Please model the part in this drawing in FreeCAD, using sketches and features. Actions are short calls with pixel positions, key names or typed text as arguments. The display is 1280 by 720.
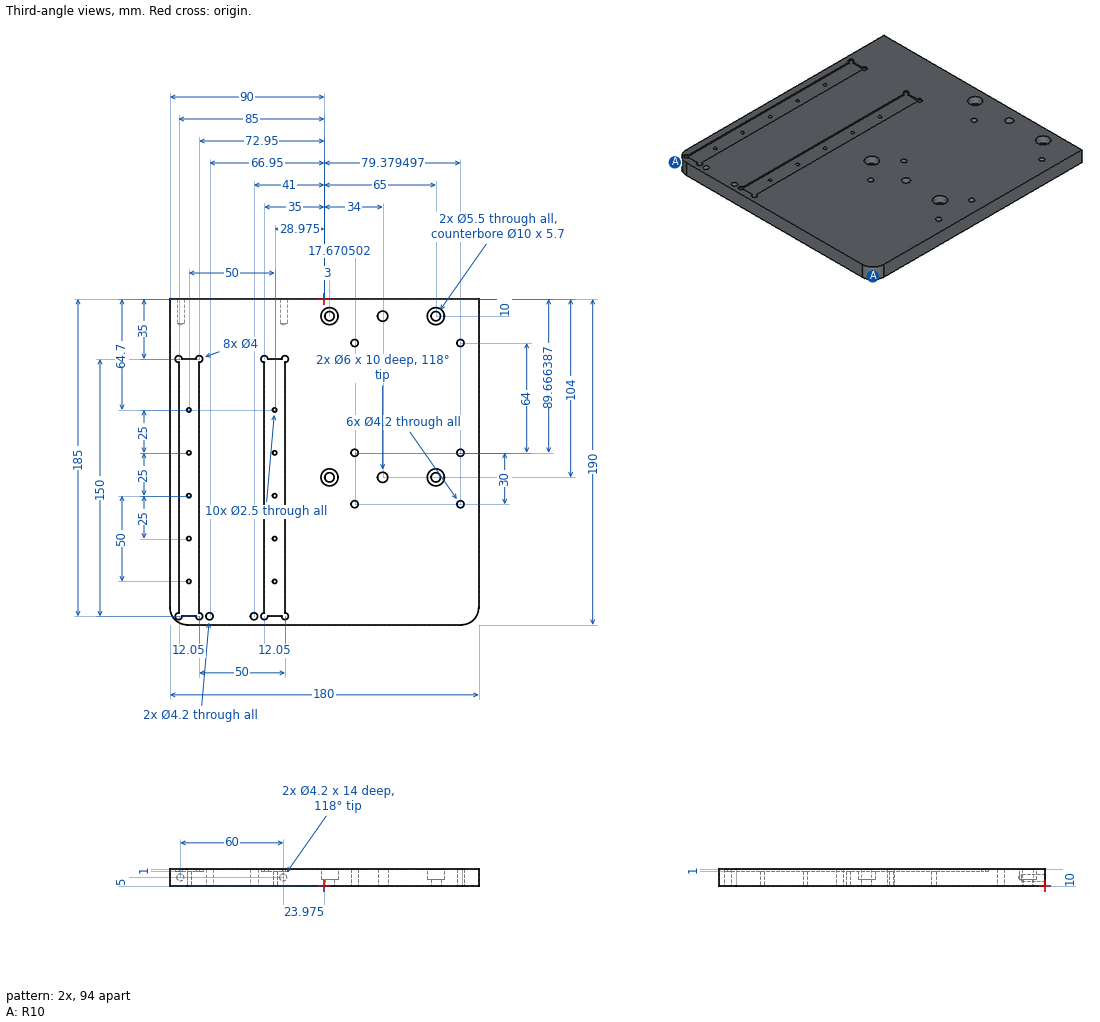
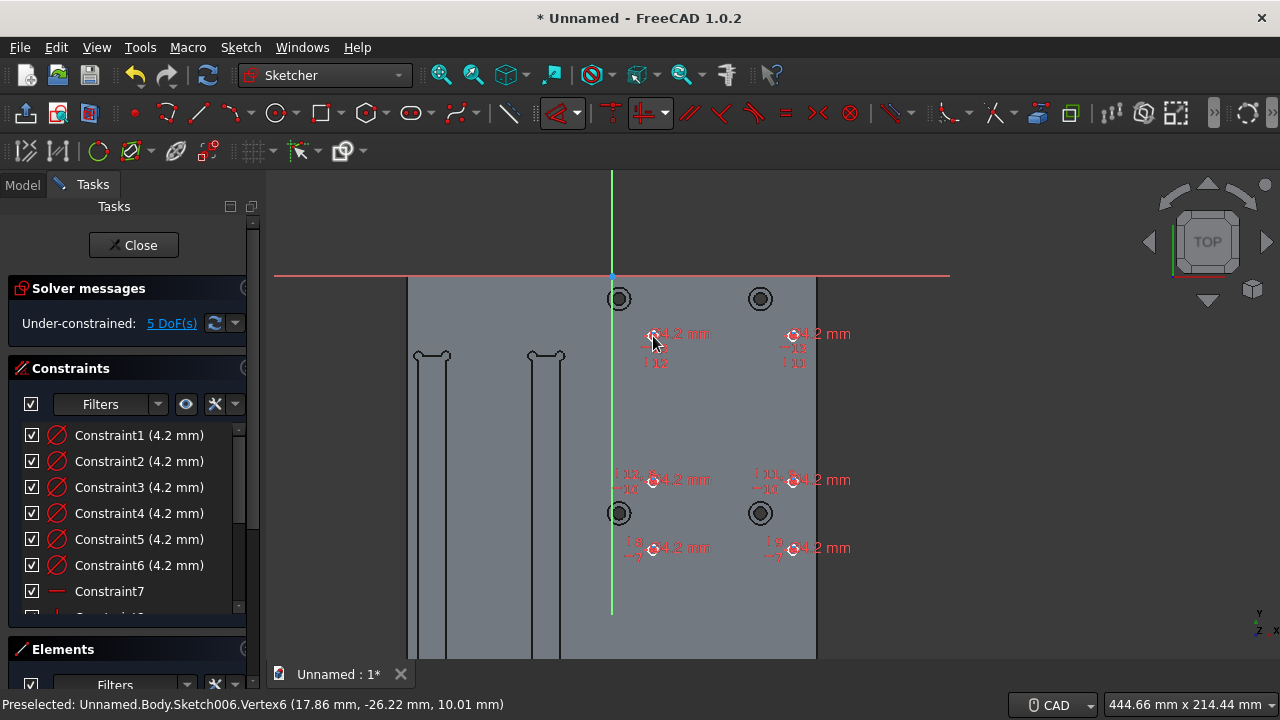
click(653, 550)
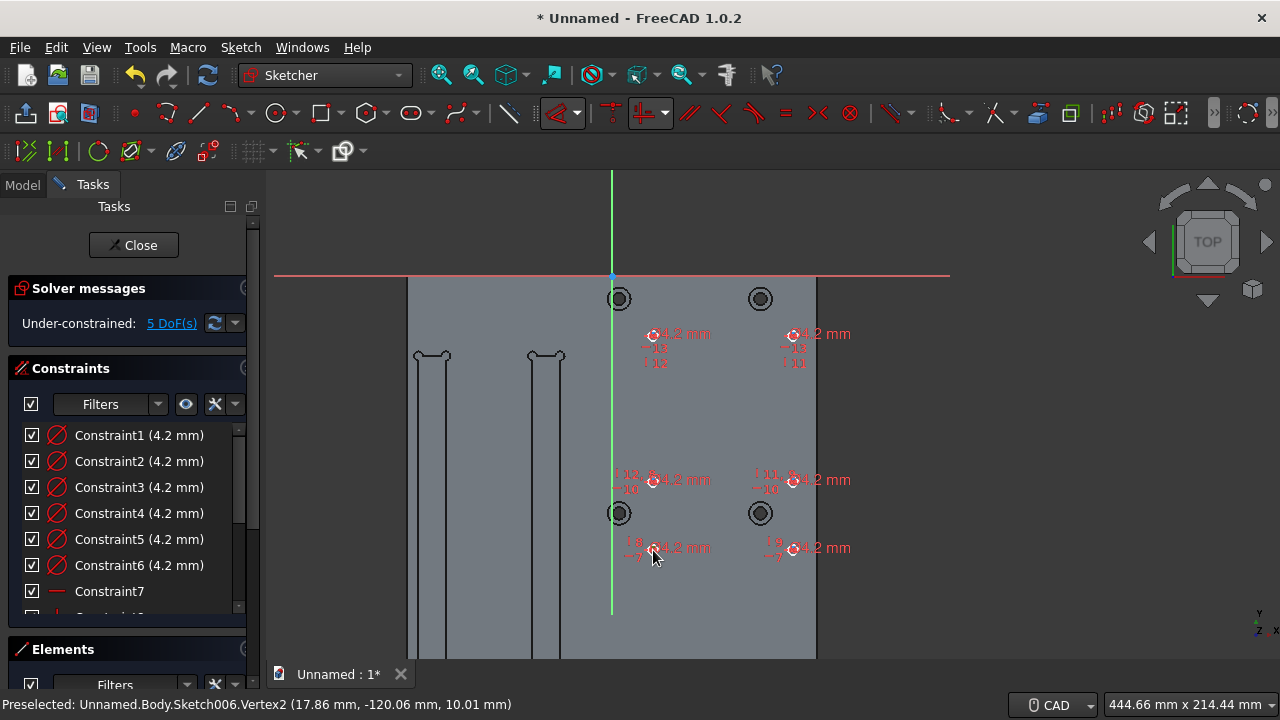
click(653, 482)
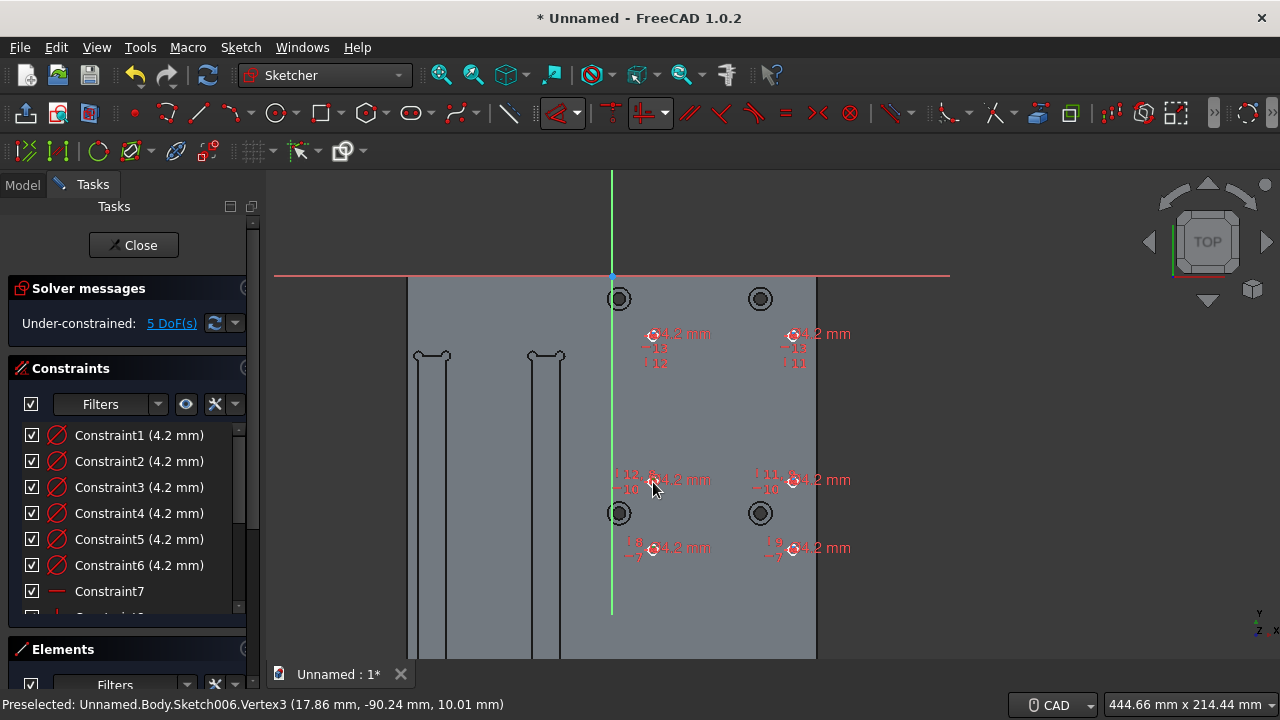
key(i)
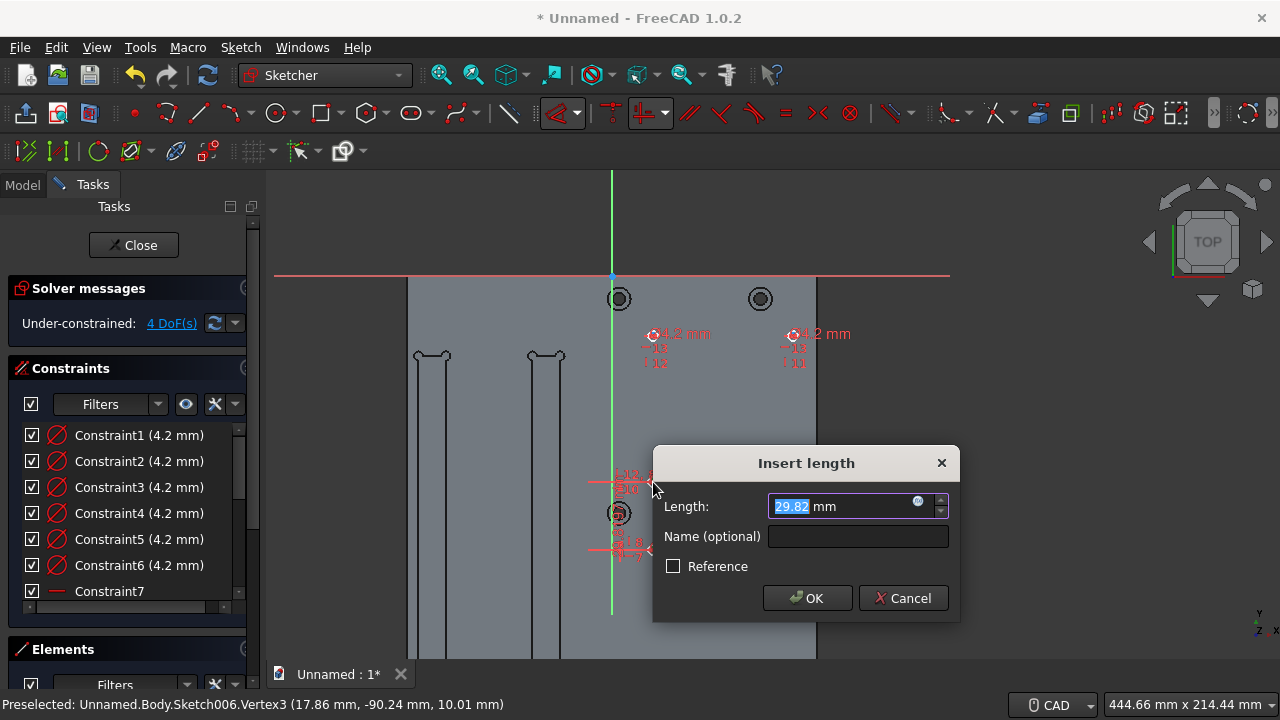
text(30)
key(Return)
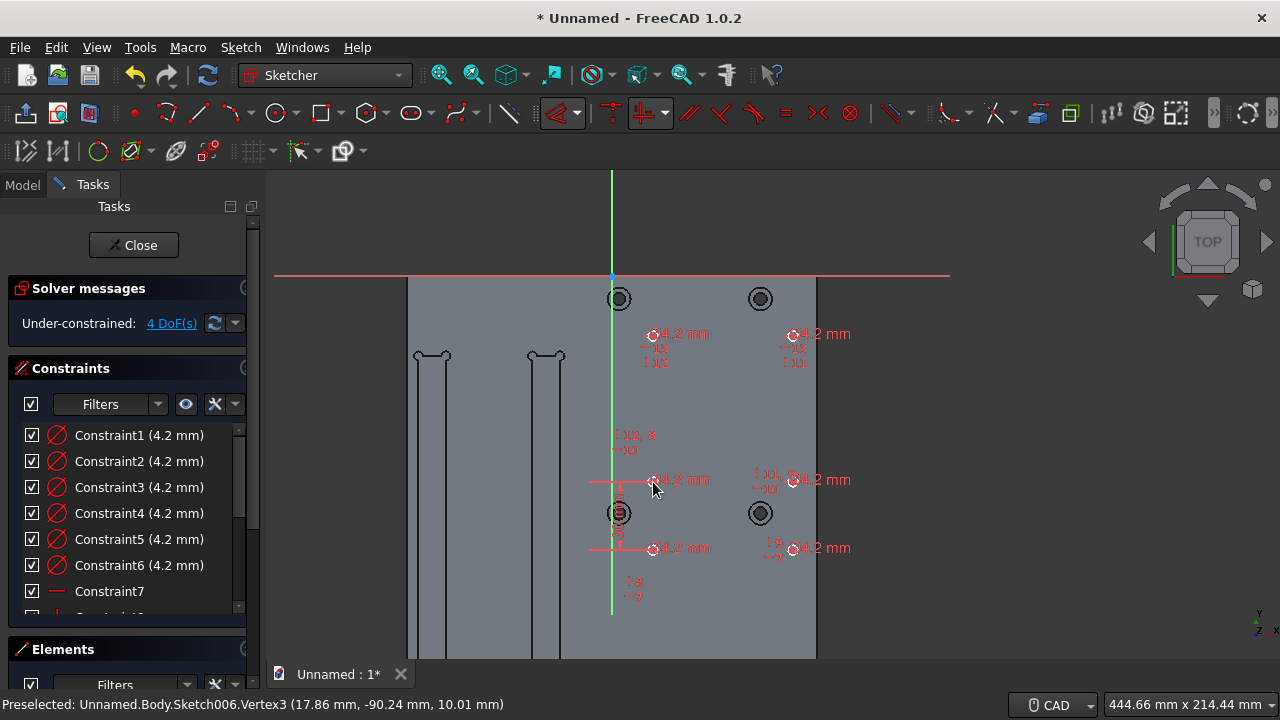
click(793, 482)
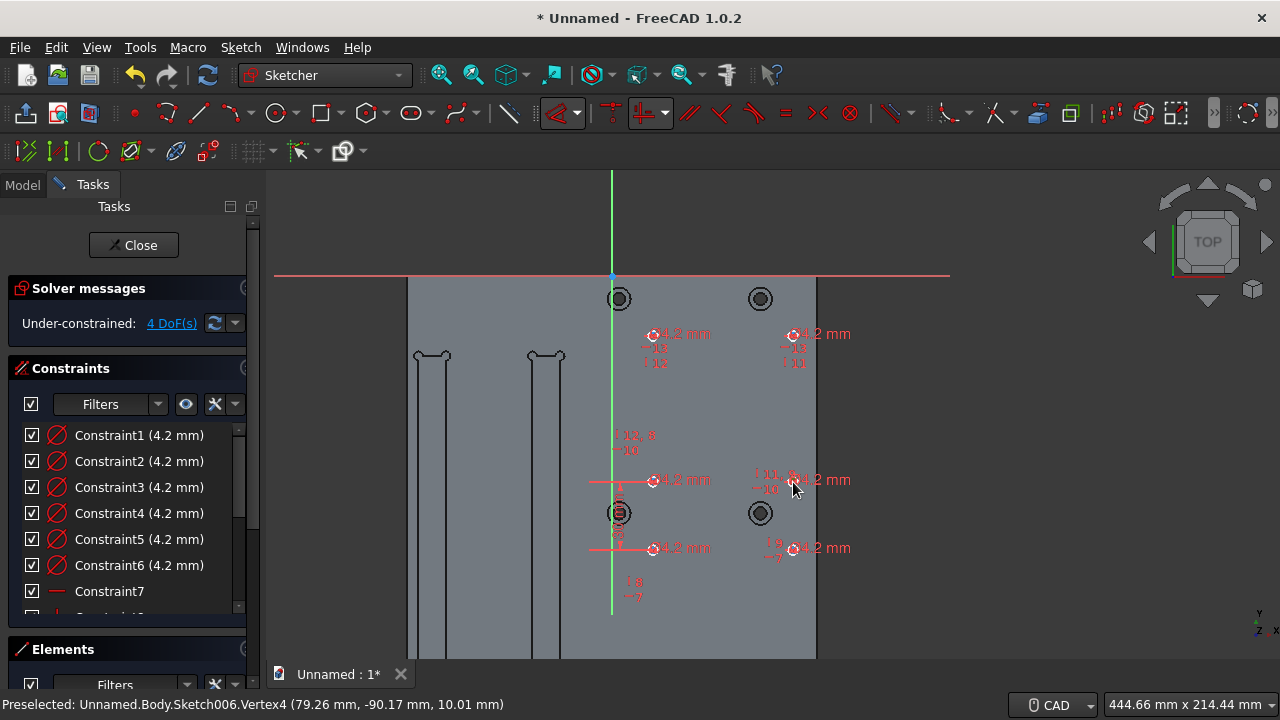
click(793, 336)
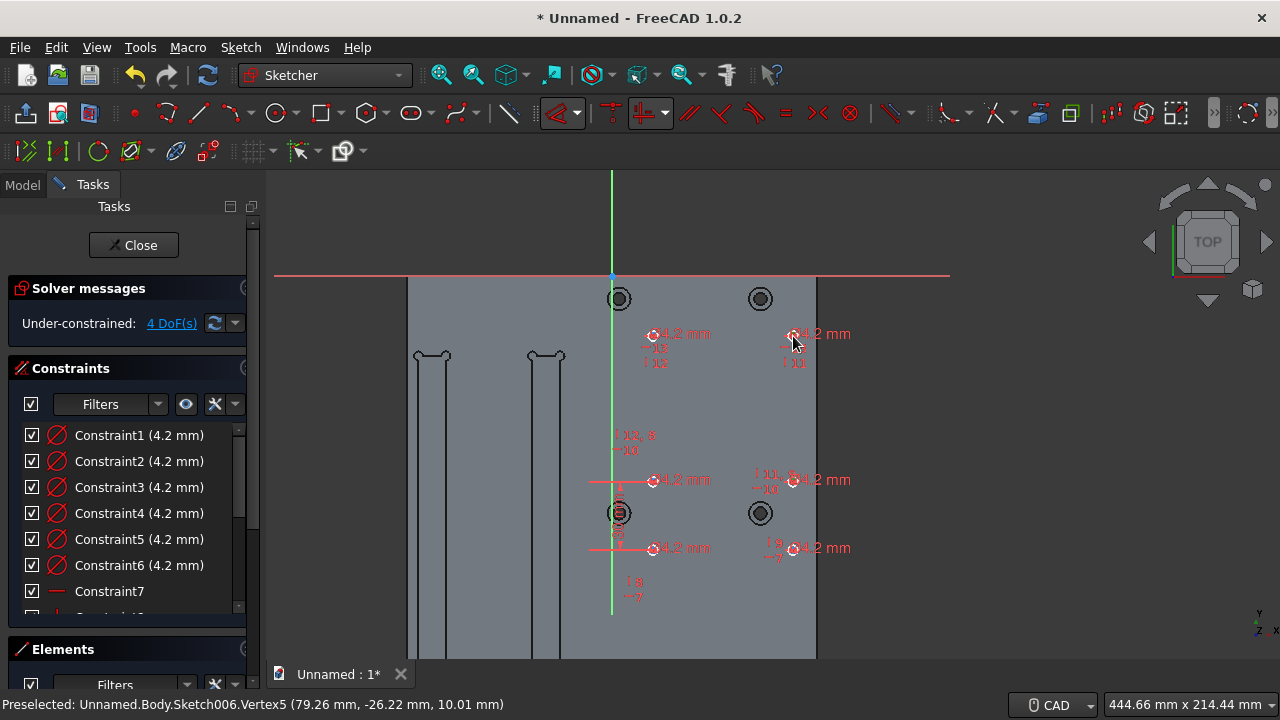
key(i)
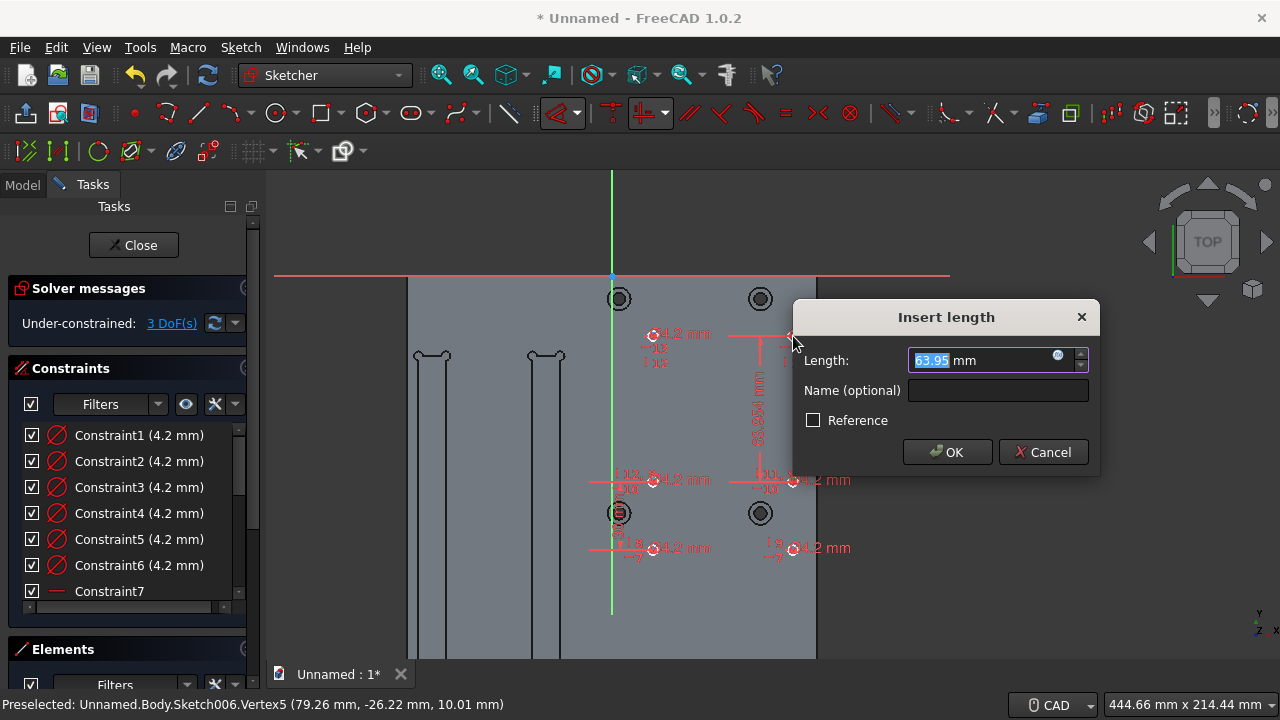
text(64)
key(Return)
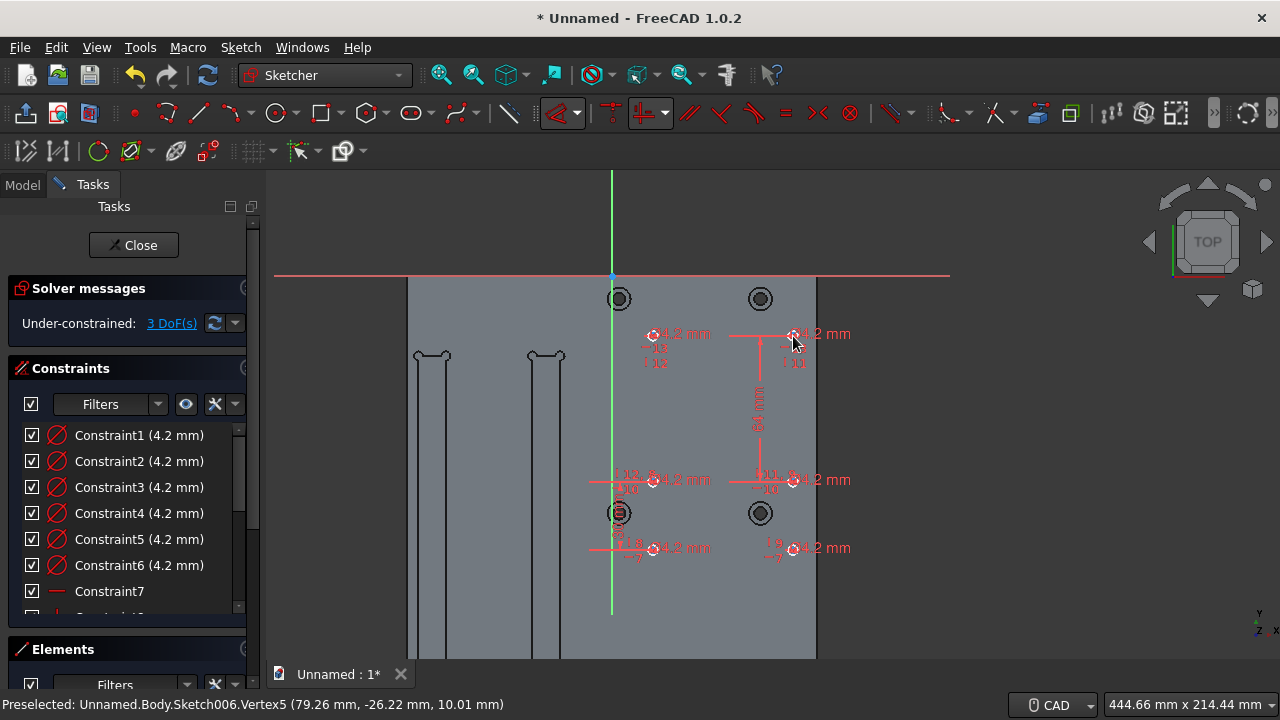
click(793, 550)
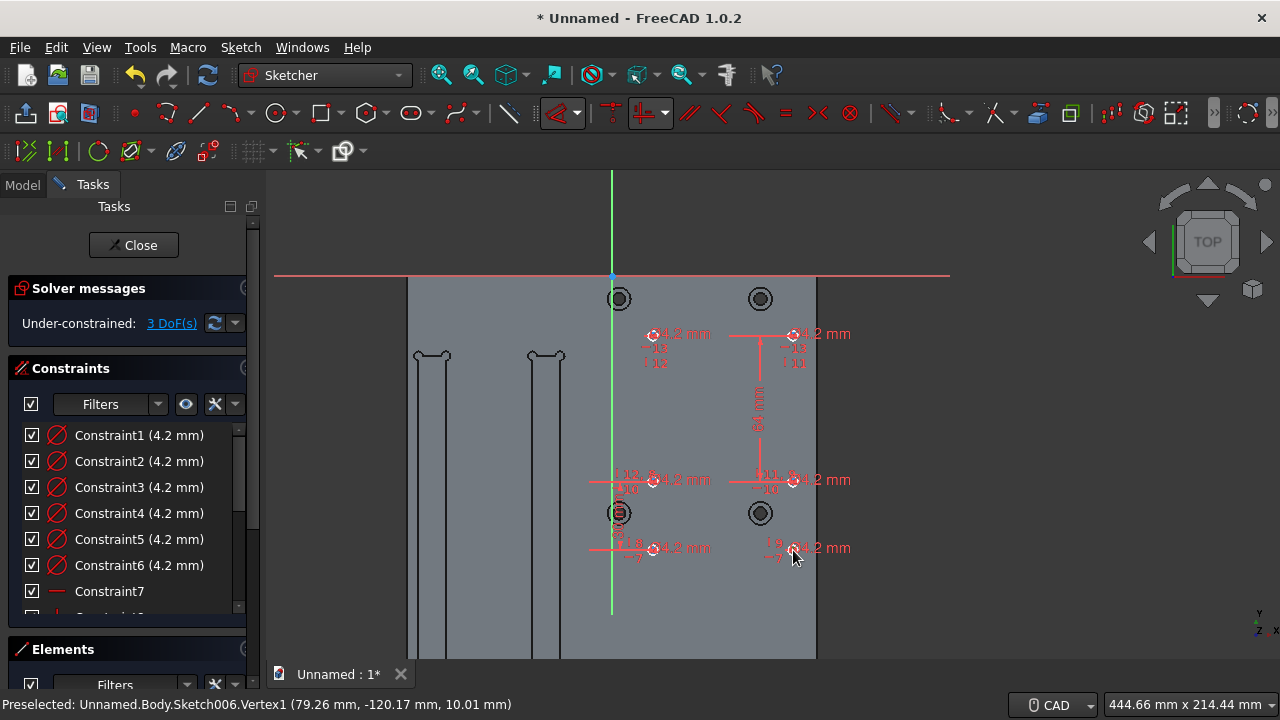
key(l)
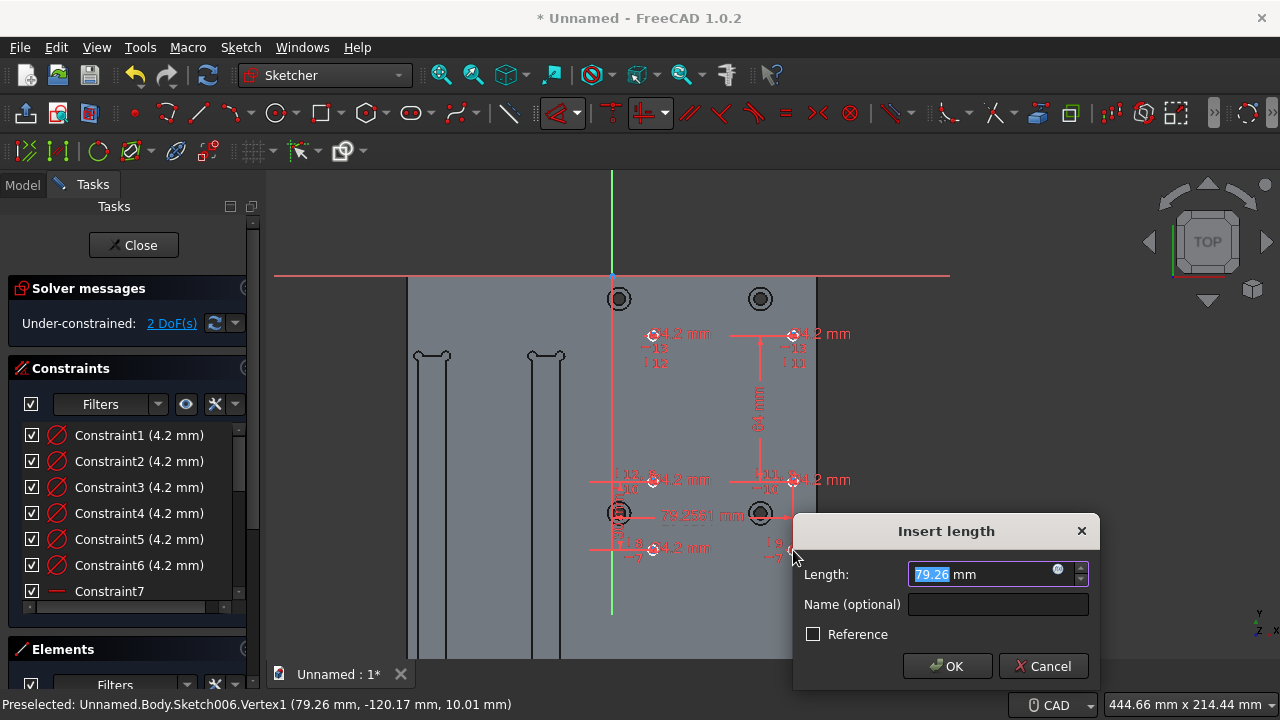
text(79.379497)
key(Return)